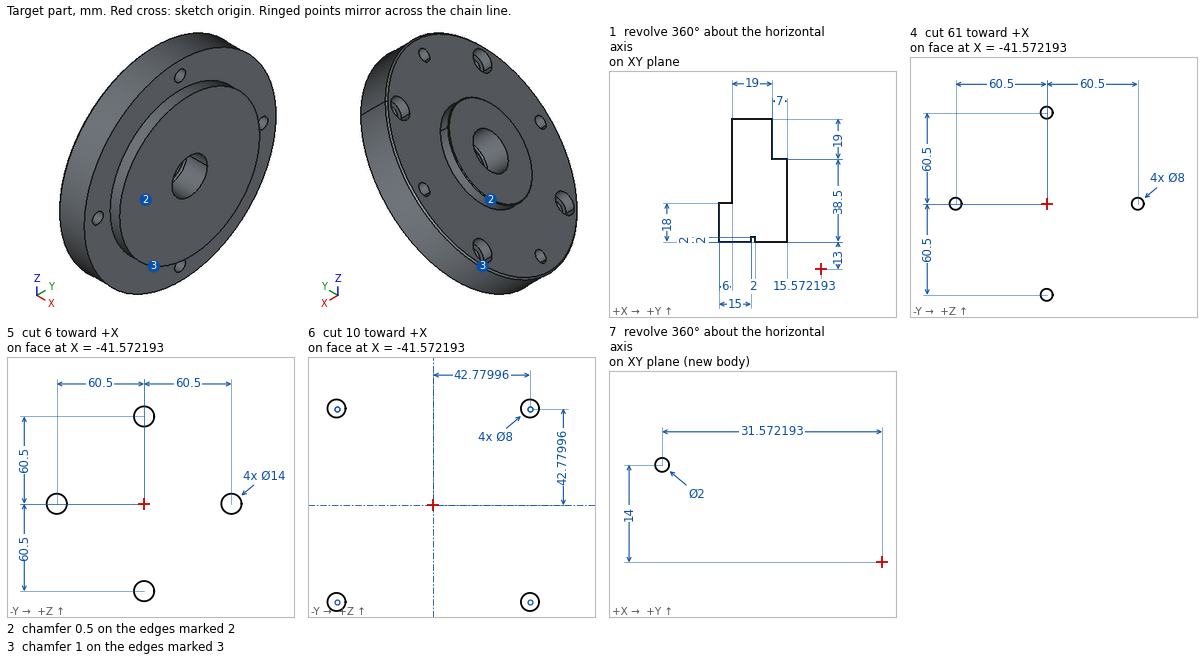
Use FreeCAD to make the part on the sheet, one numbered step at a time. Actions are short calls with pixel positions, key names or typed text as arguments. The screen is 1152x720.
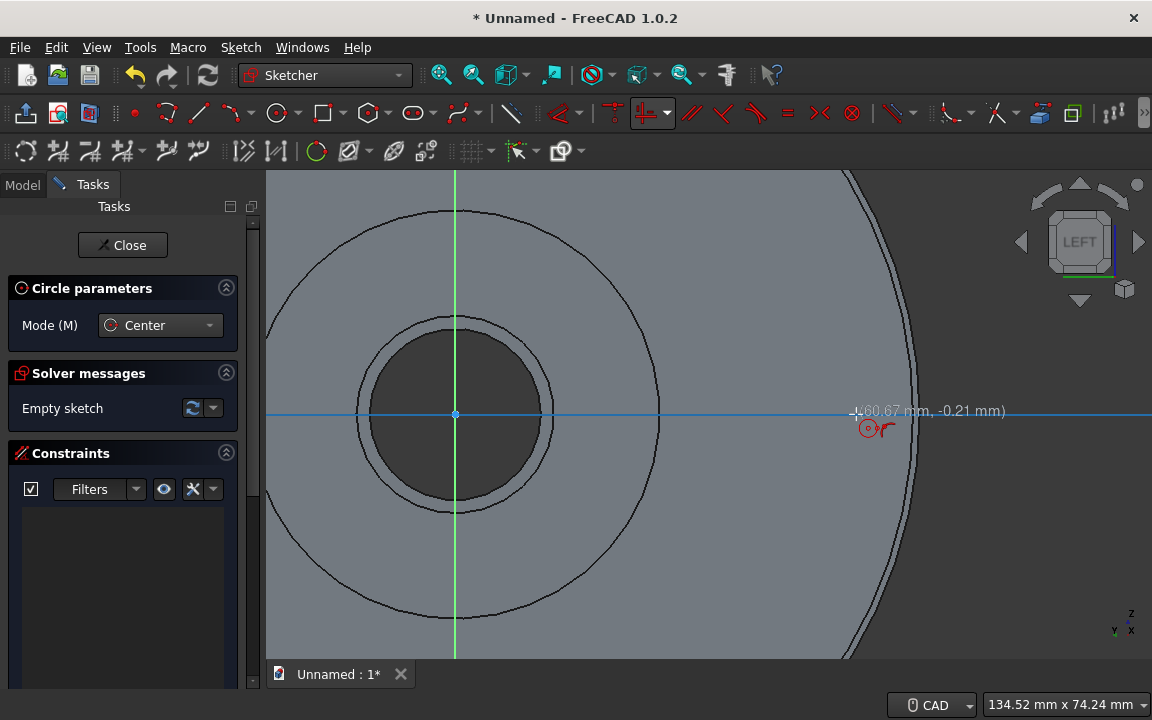
click(854, 414)
move(872, 396)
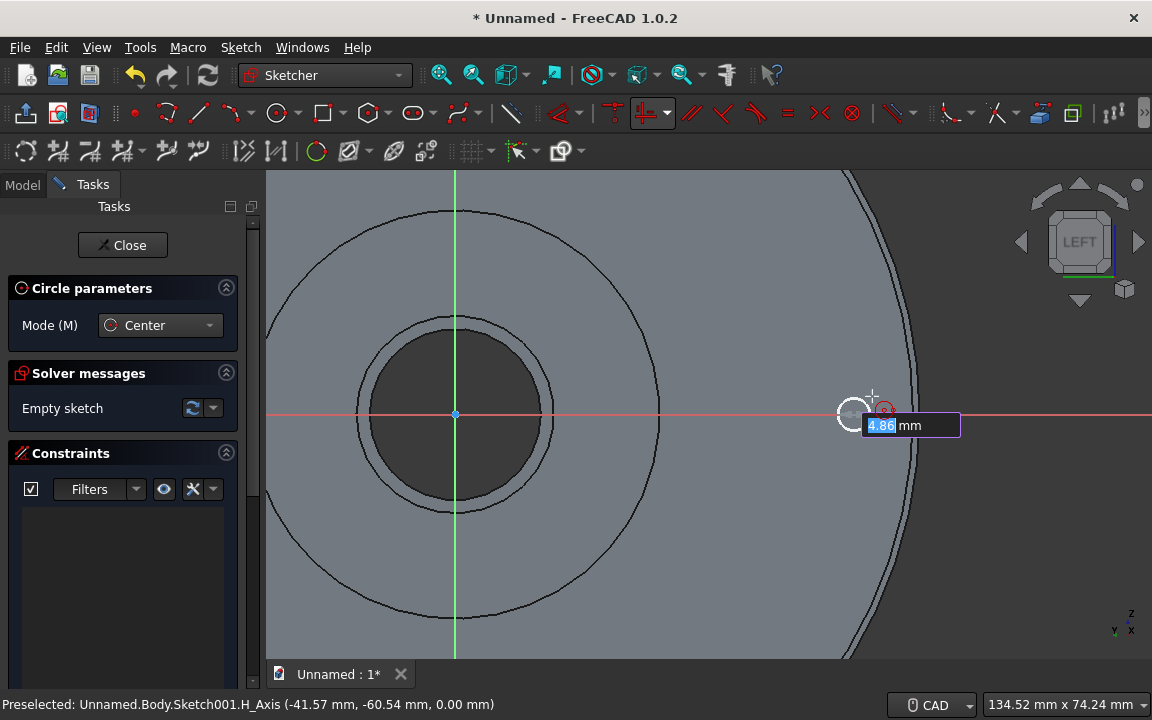
text(8)
key(Return)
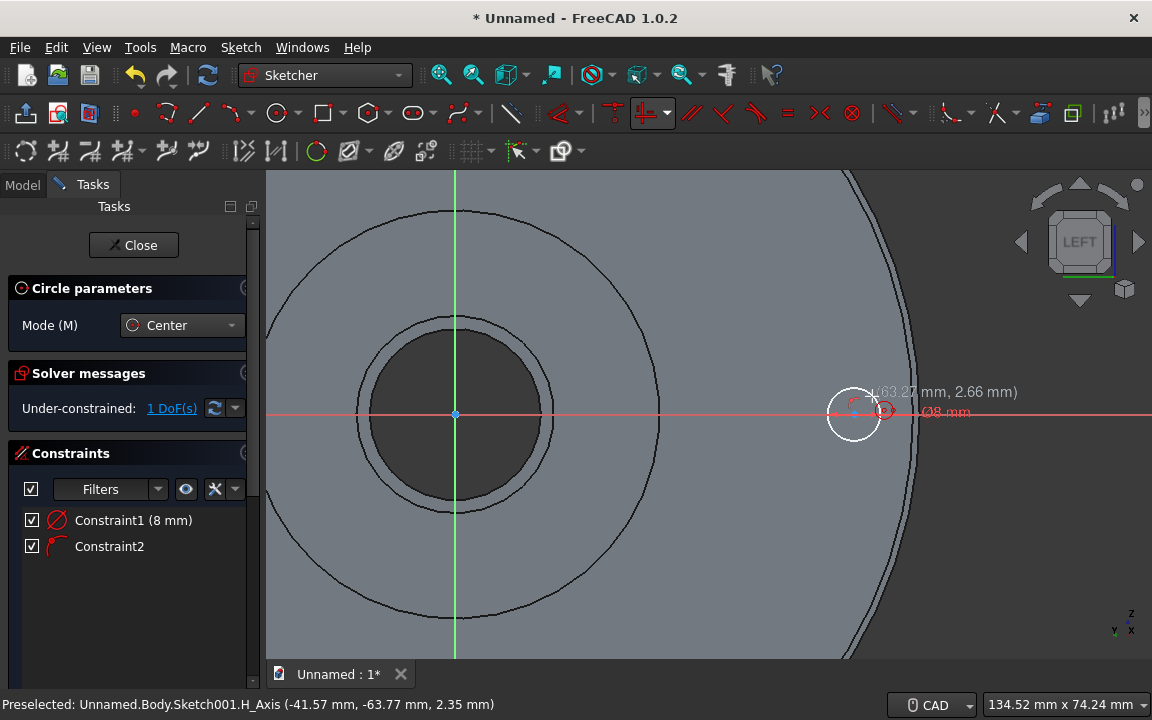
scroll(748, 414, down, 5)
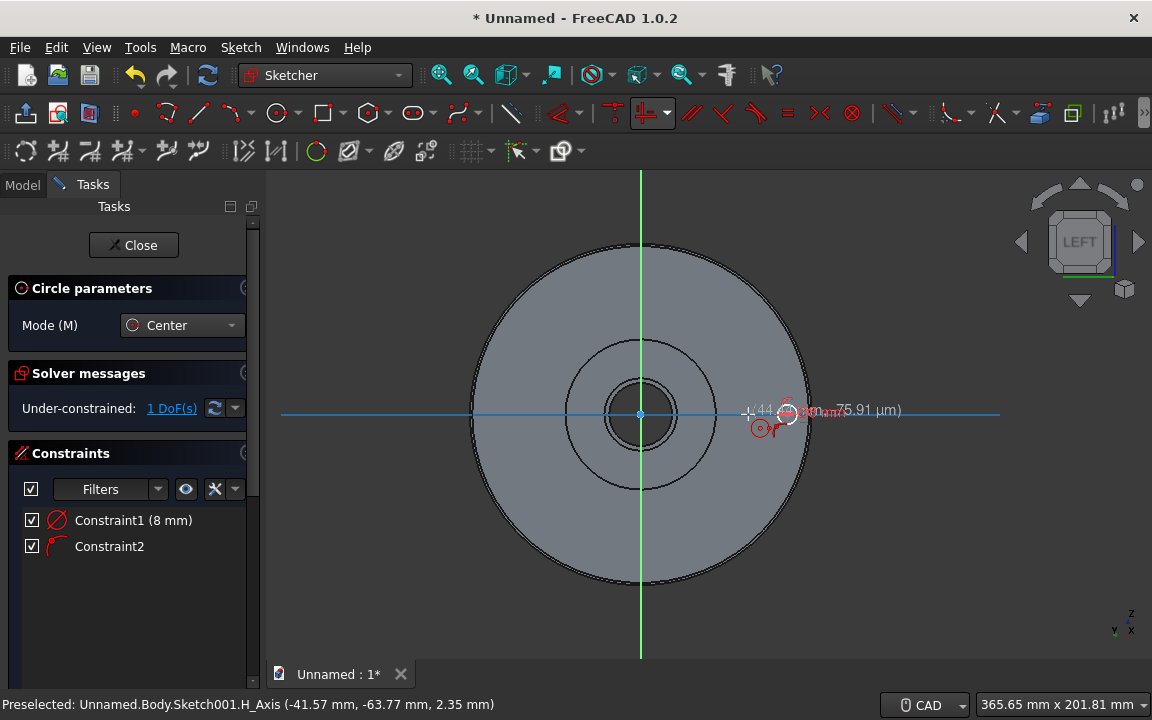
scroll(641, 561, up, 5)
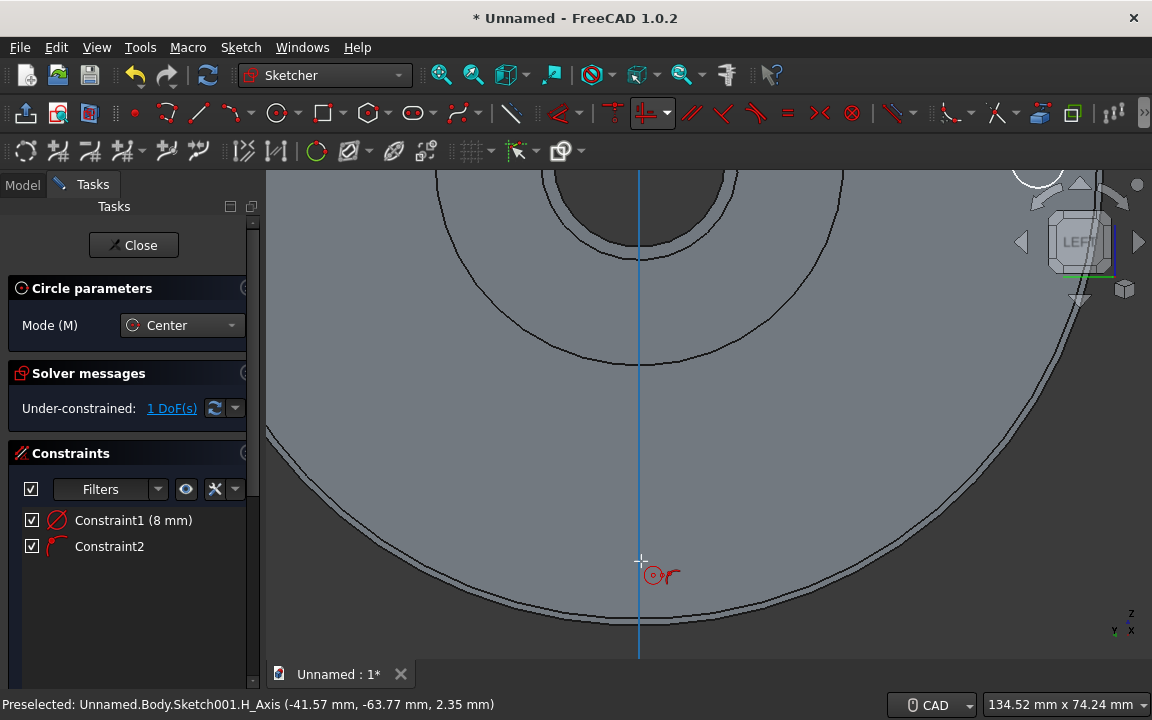
click(639, 560)
move(658, 541)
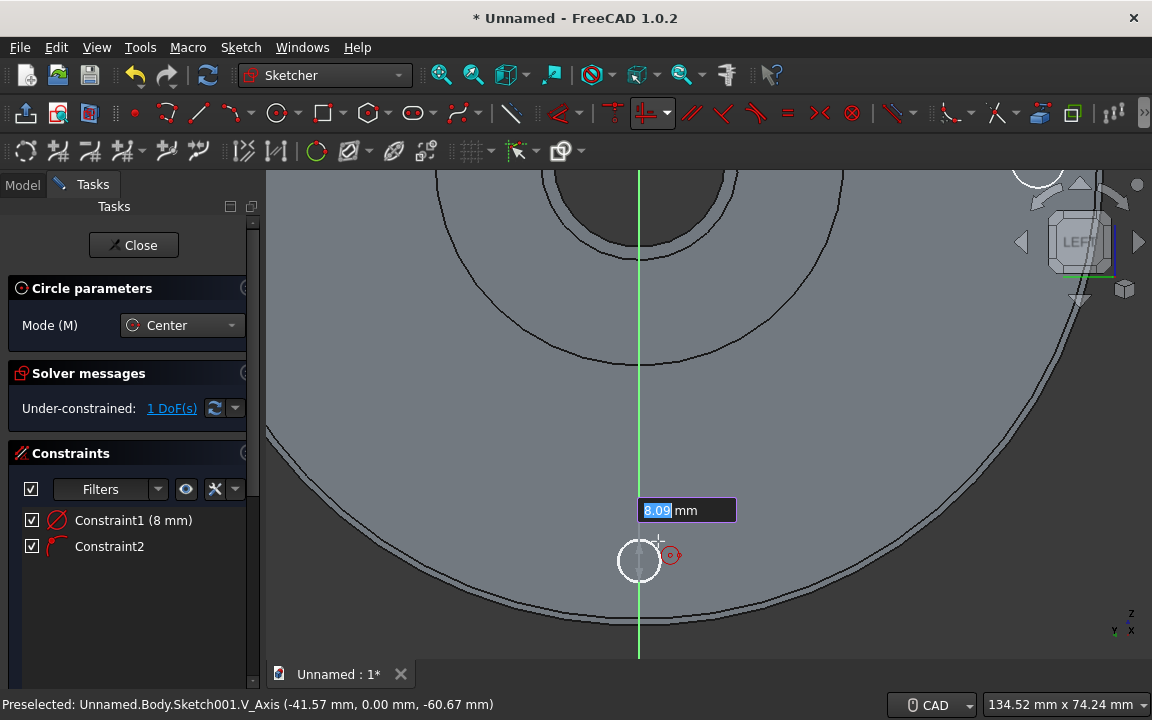
text(8)
key(Return)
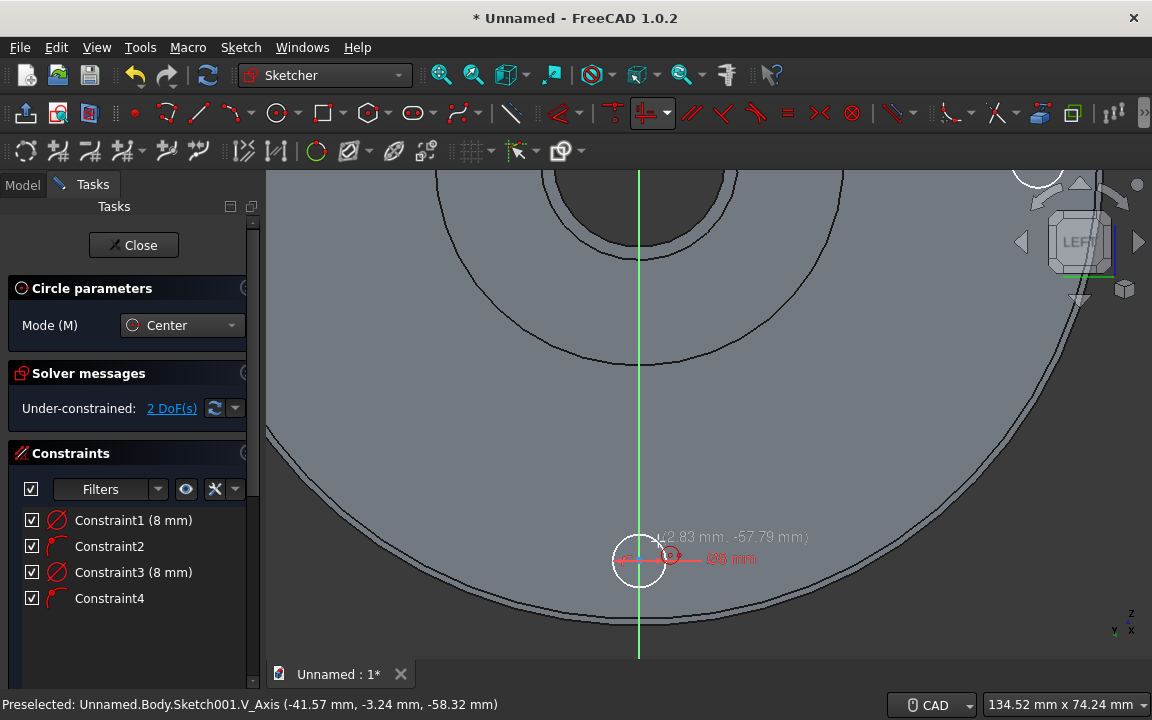
scroll(641, 562, down, 5)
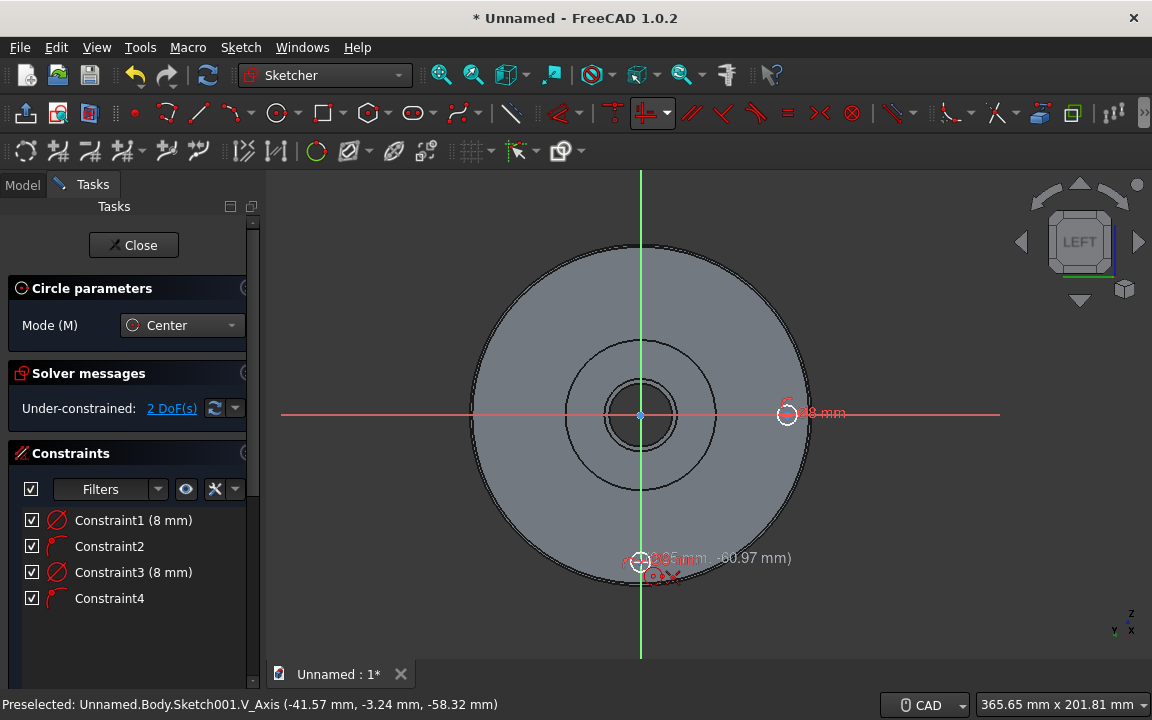
scroll(494, 415, up, 5)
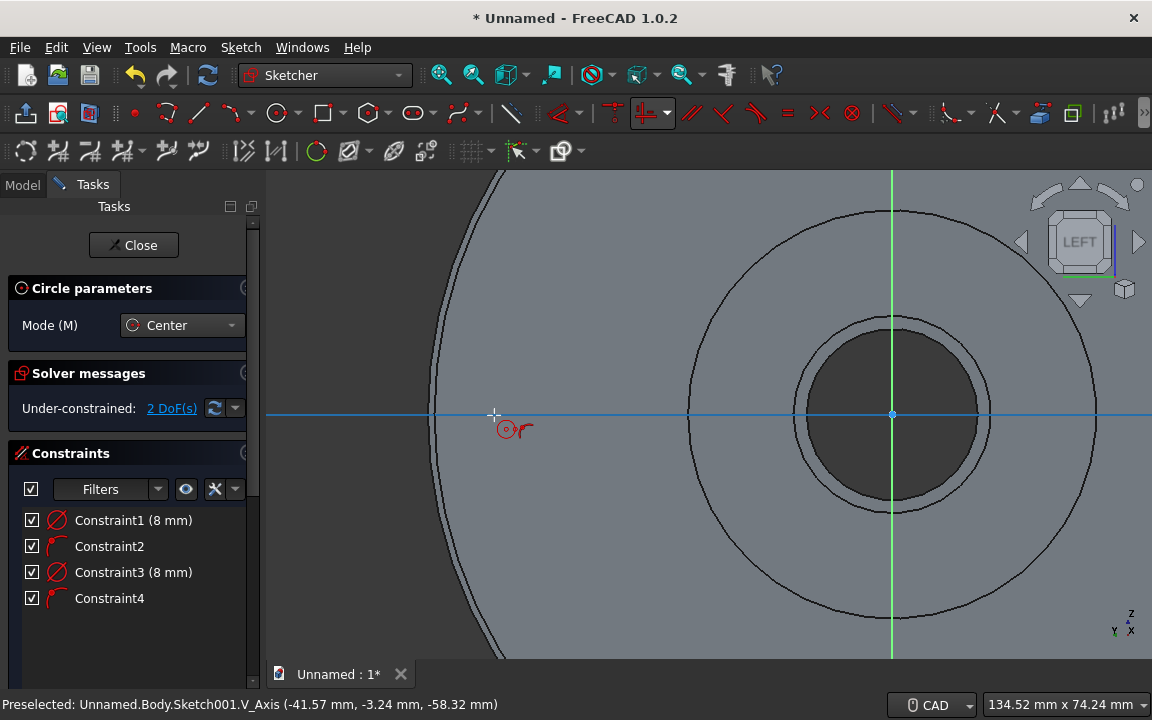
click(494, 415)
move(512, 396)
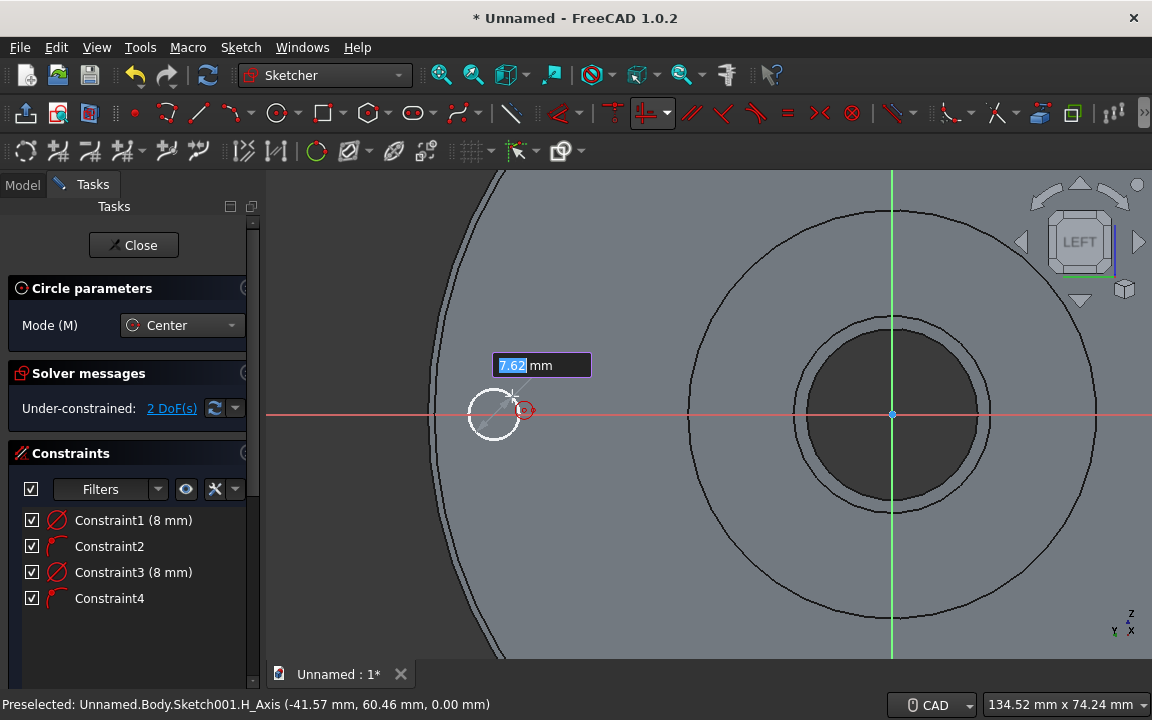
text(8)
key(Return)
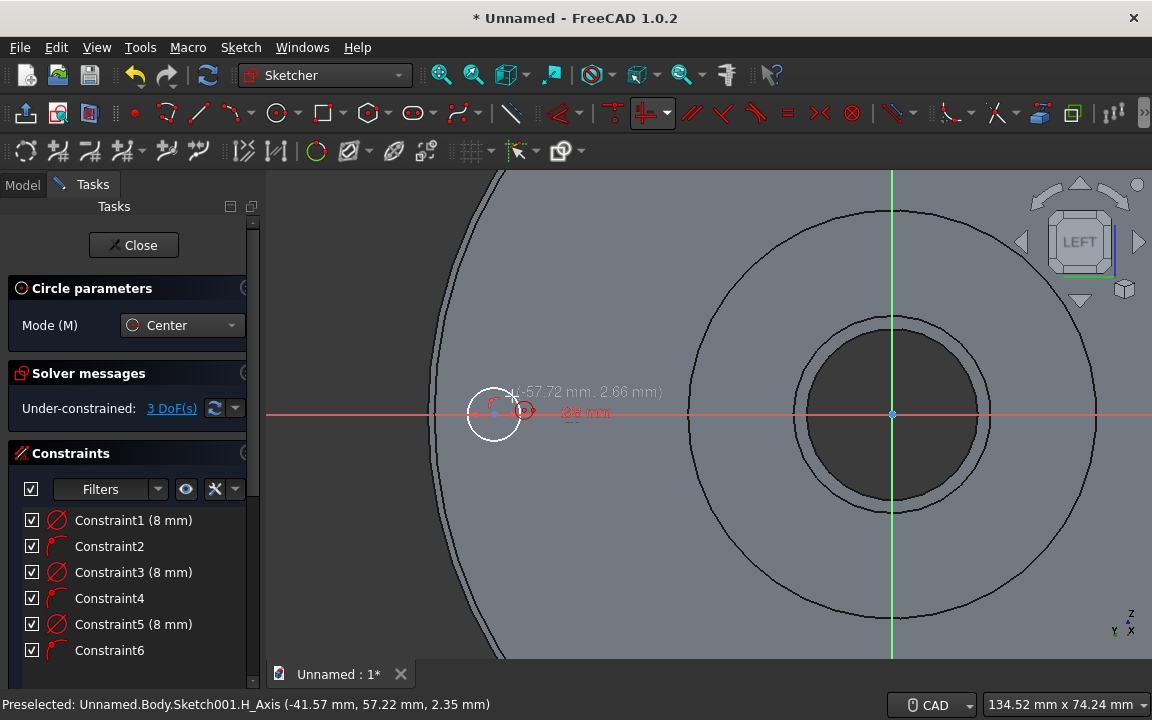
scroll(494, 414, down, 5)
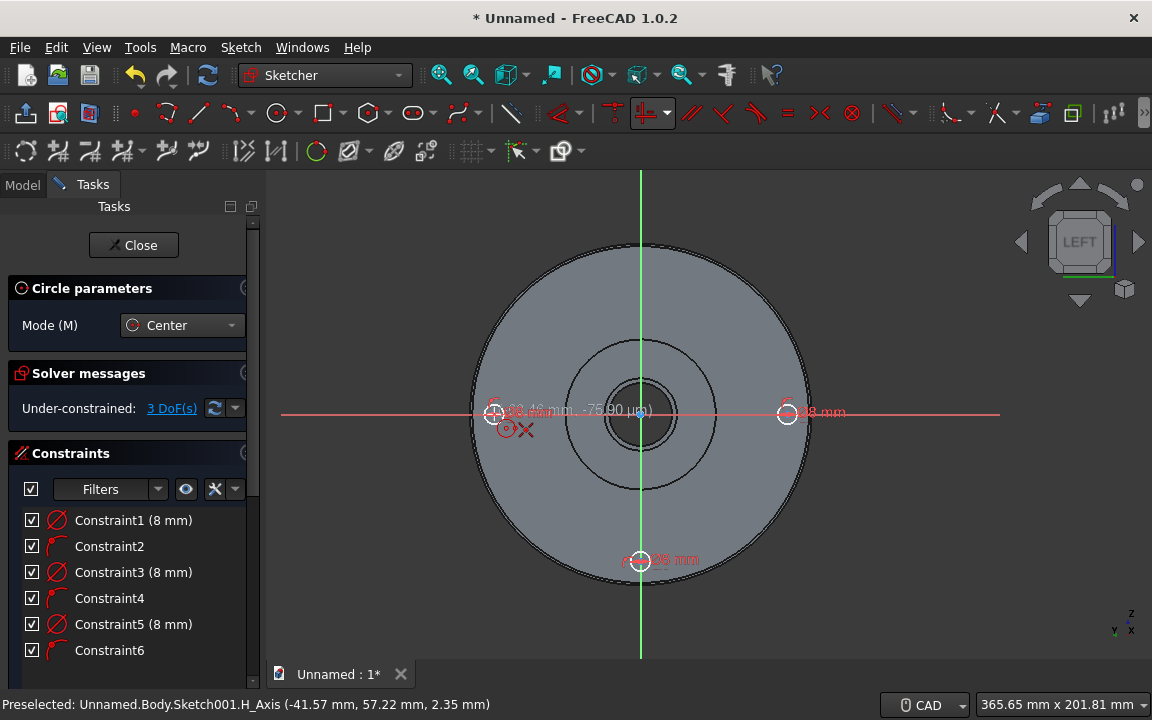
scroll(641, 268, up, 5)